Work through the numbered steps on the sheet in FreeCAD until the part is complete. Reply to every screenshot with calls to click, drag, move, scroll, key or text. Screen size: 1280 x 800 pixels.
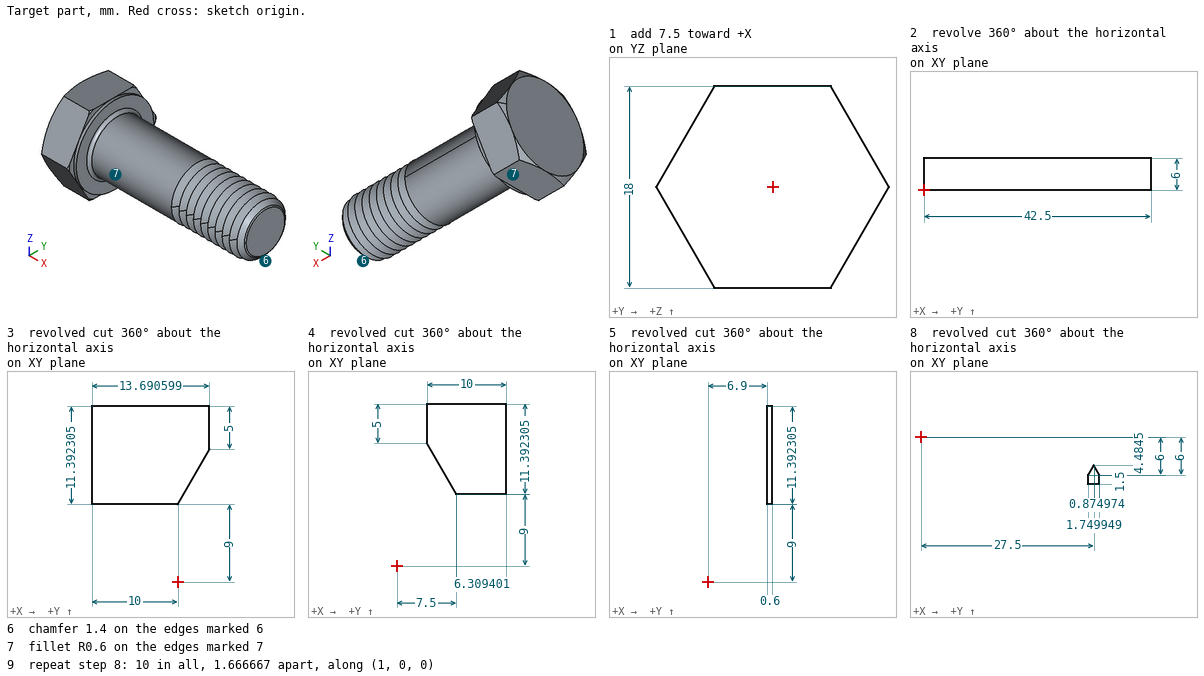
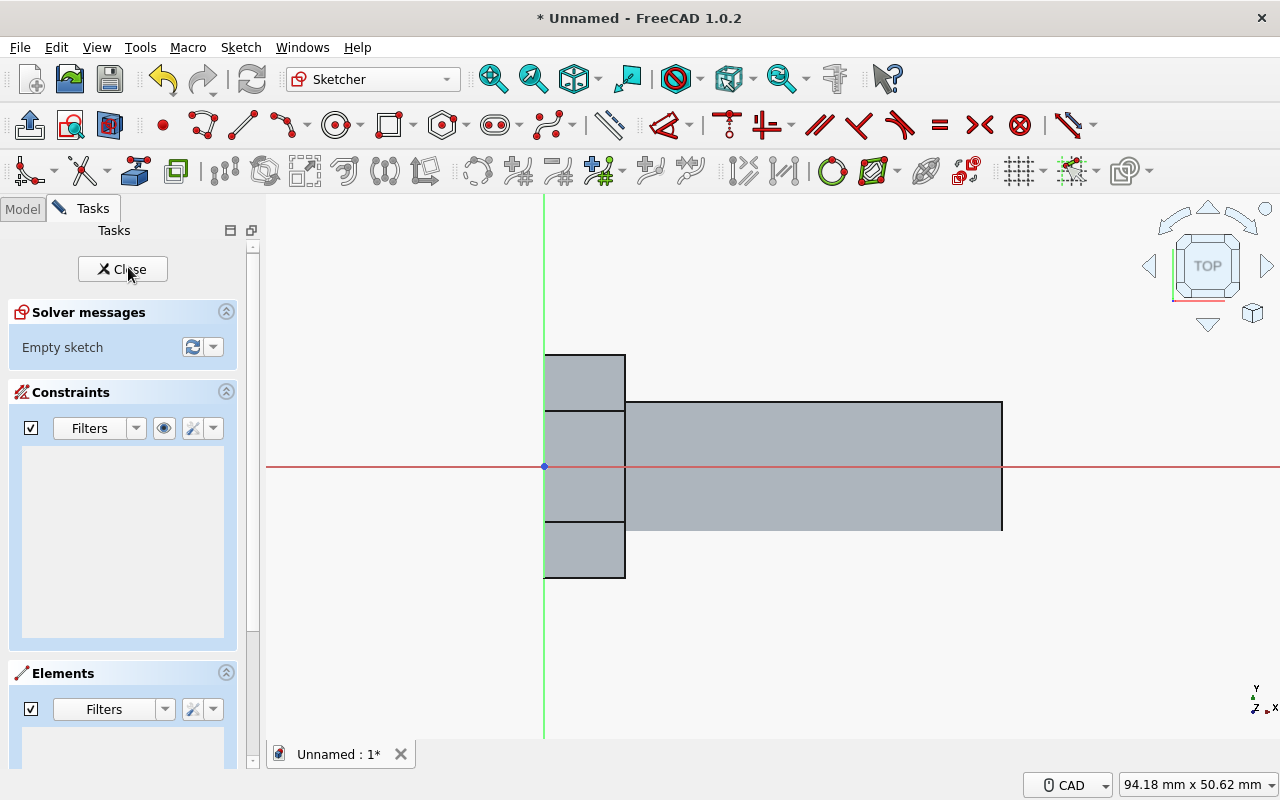
scroll(294, 222, up, 2)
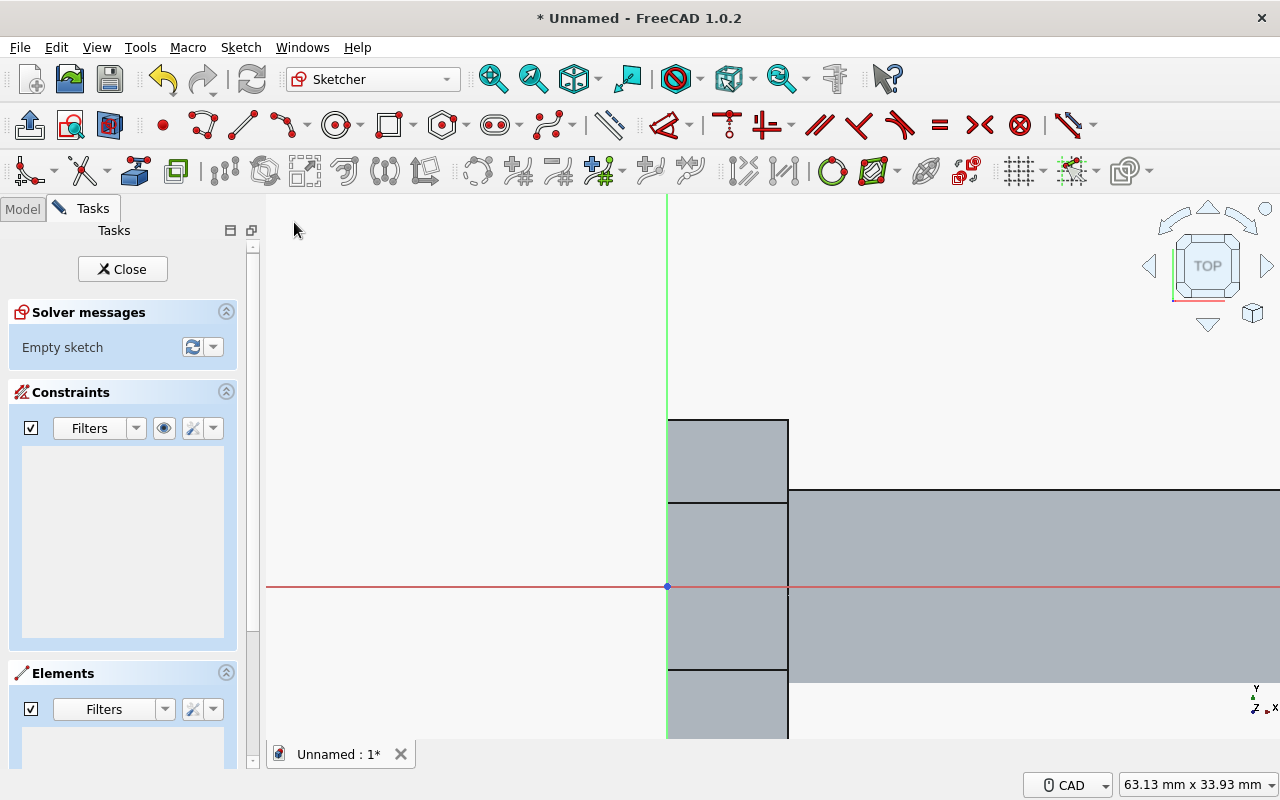
click(204, 126)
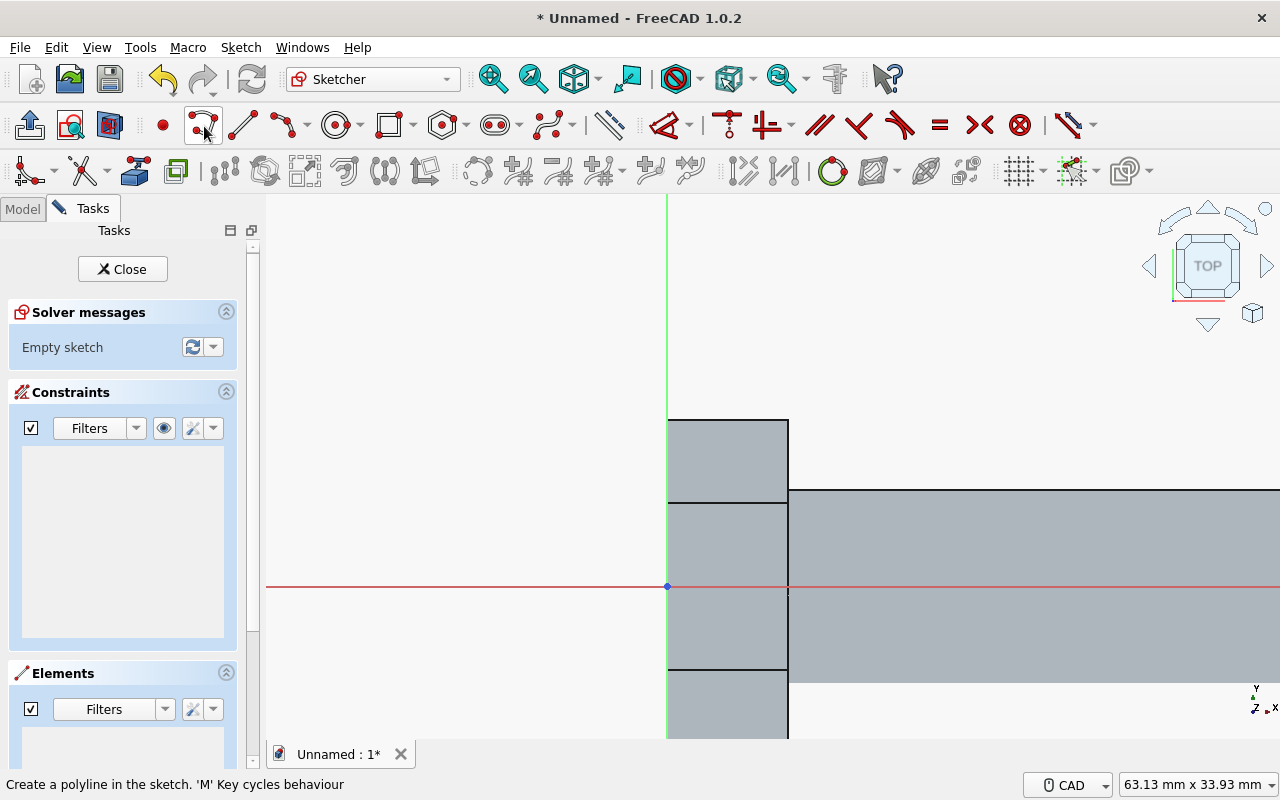
click(667, 442)
click(727, 339)
click(727, 259)
click(507, 259)
click(507, 442)
click(667, 443)
key(Escape)
key(Escape)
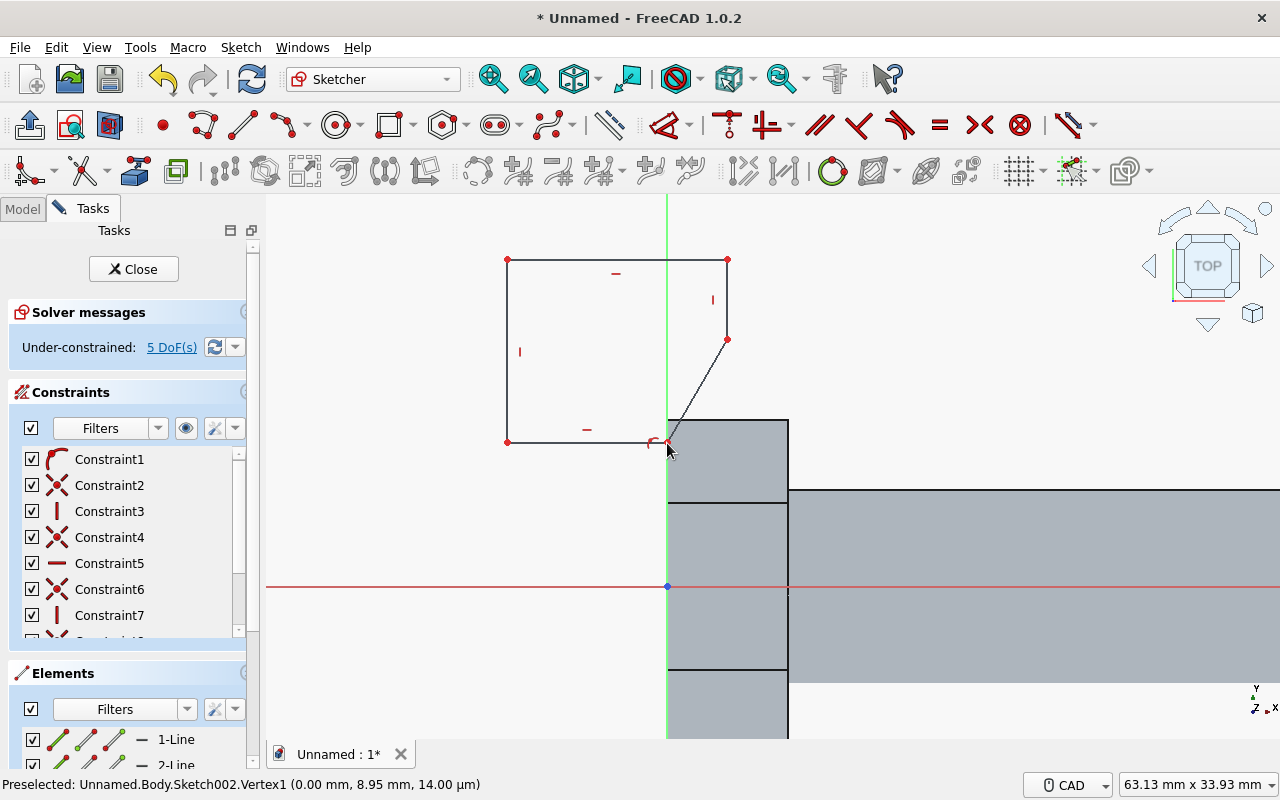
click(727, 316)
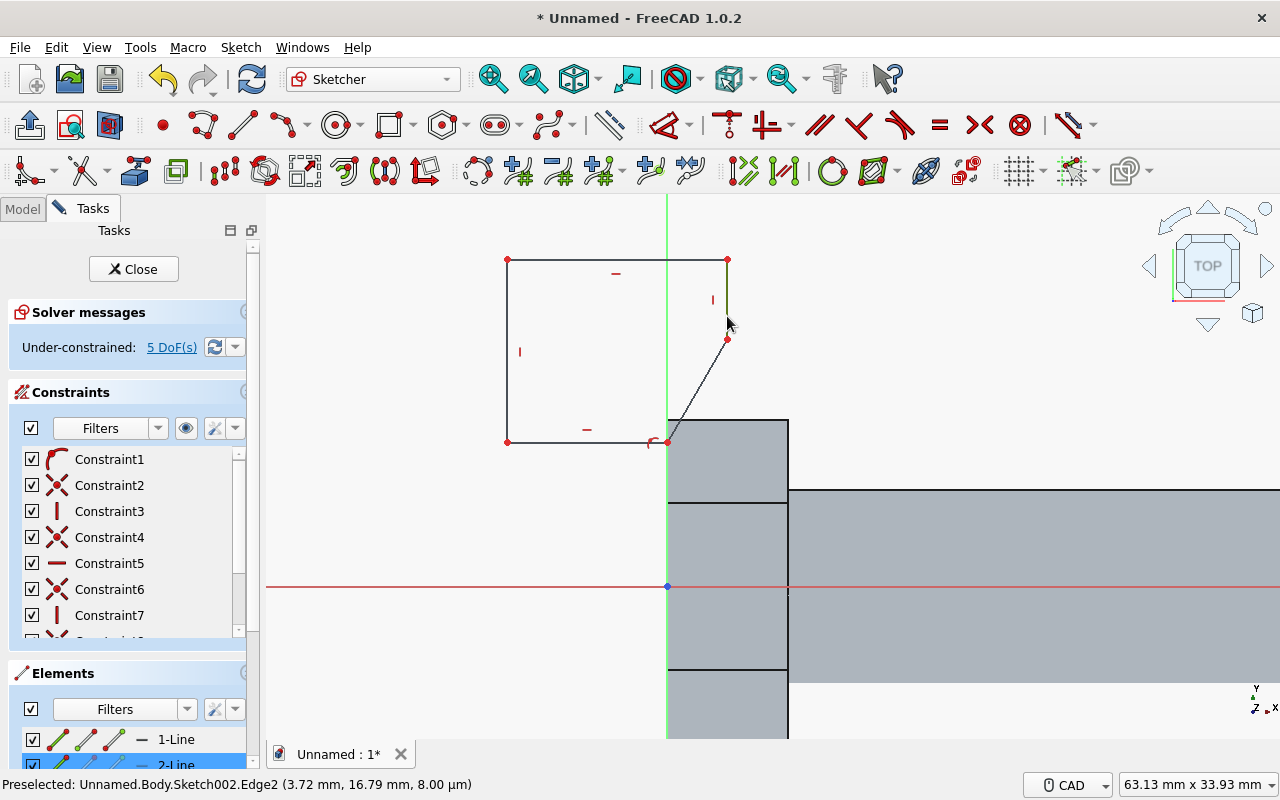
key(i)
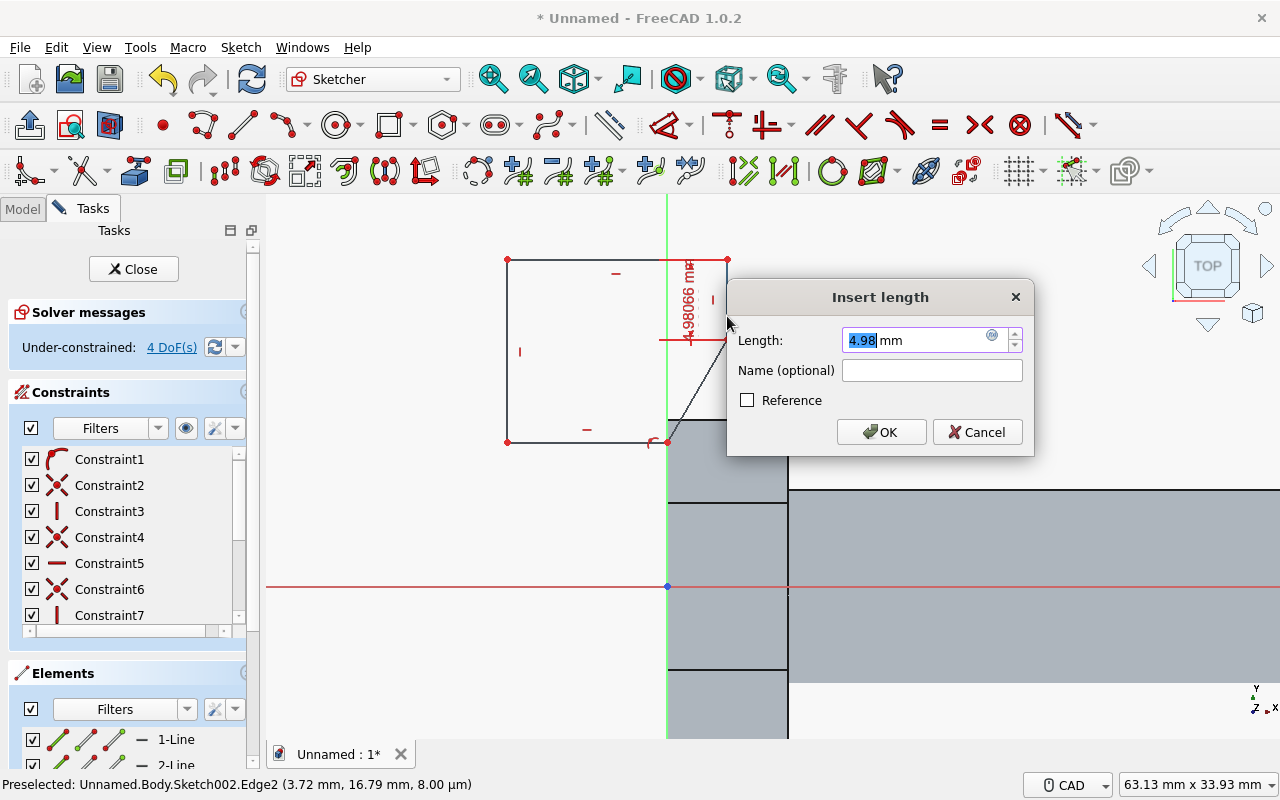
text(5)
key(Return)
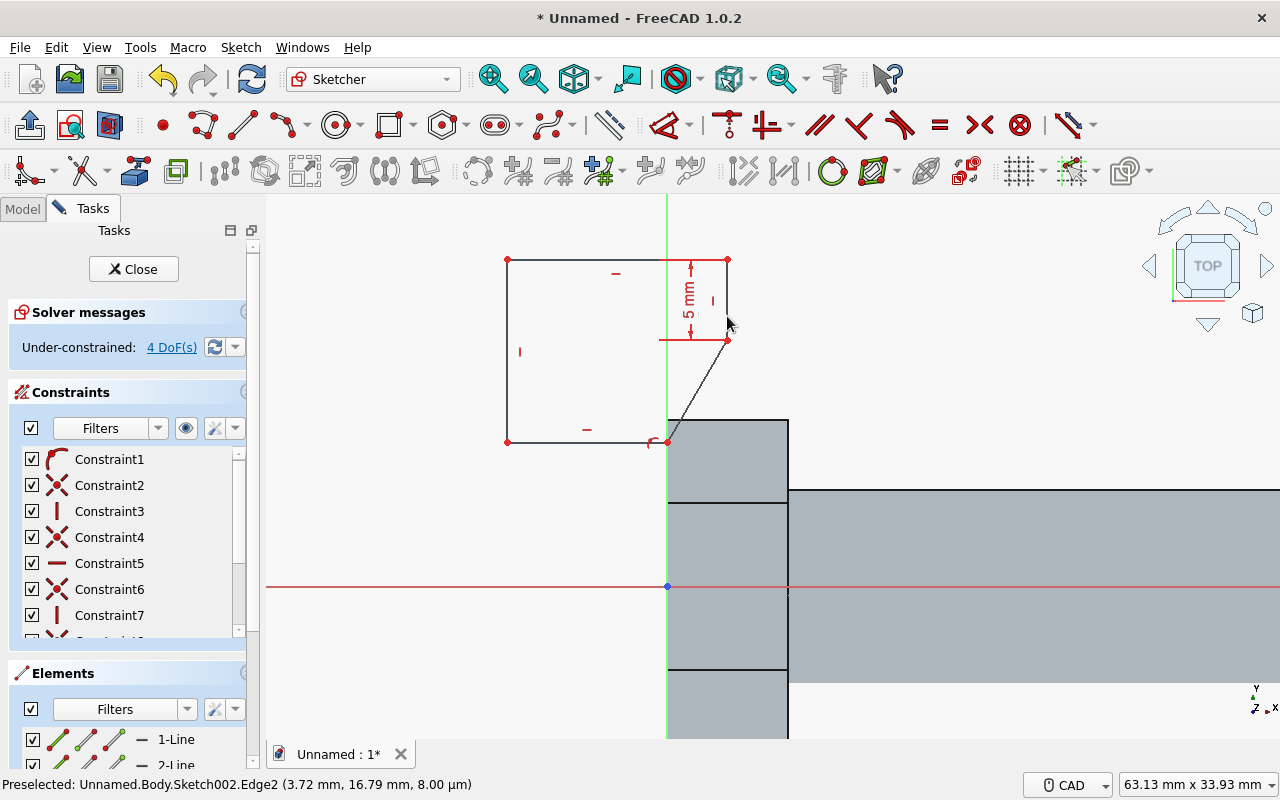
click(555, 443)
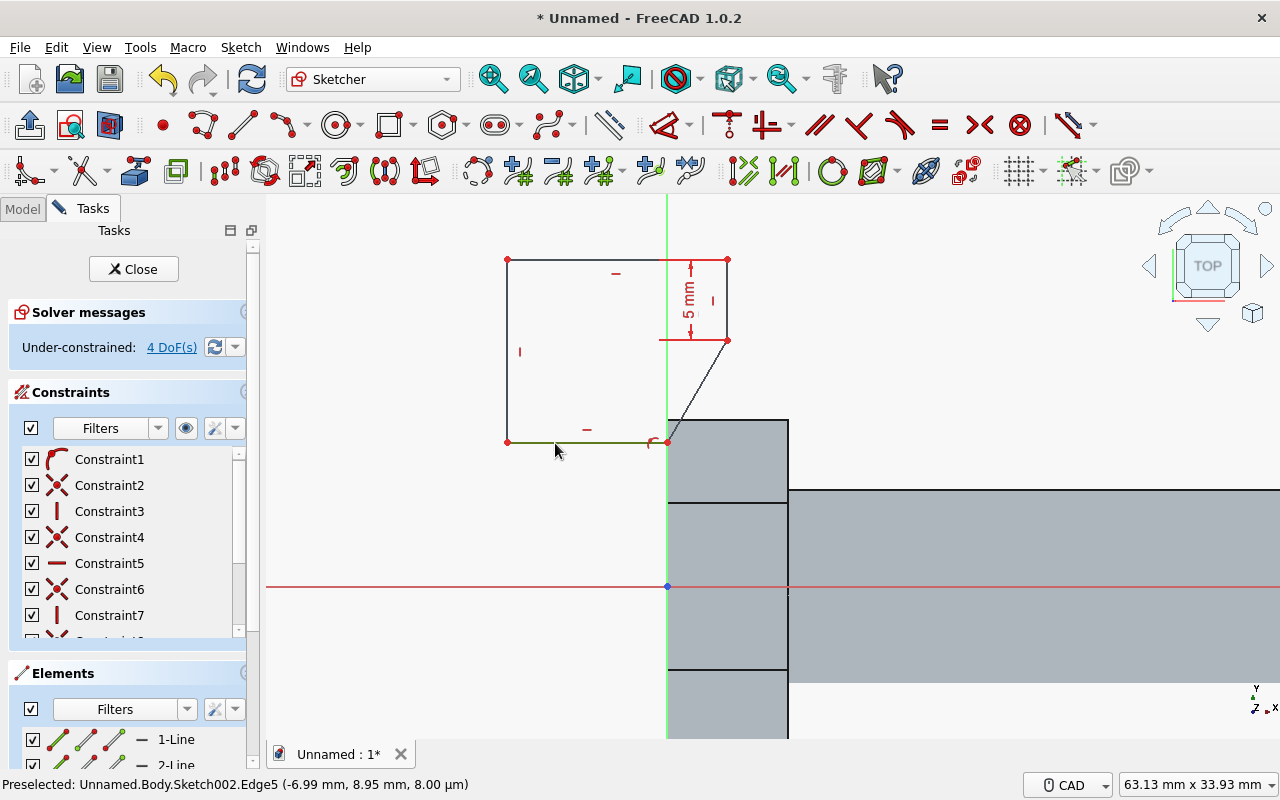
key(l)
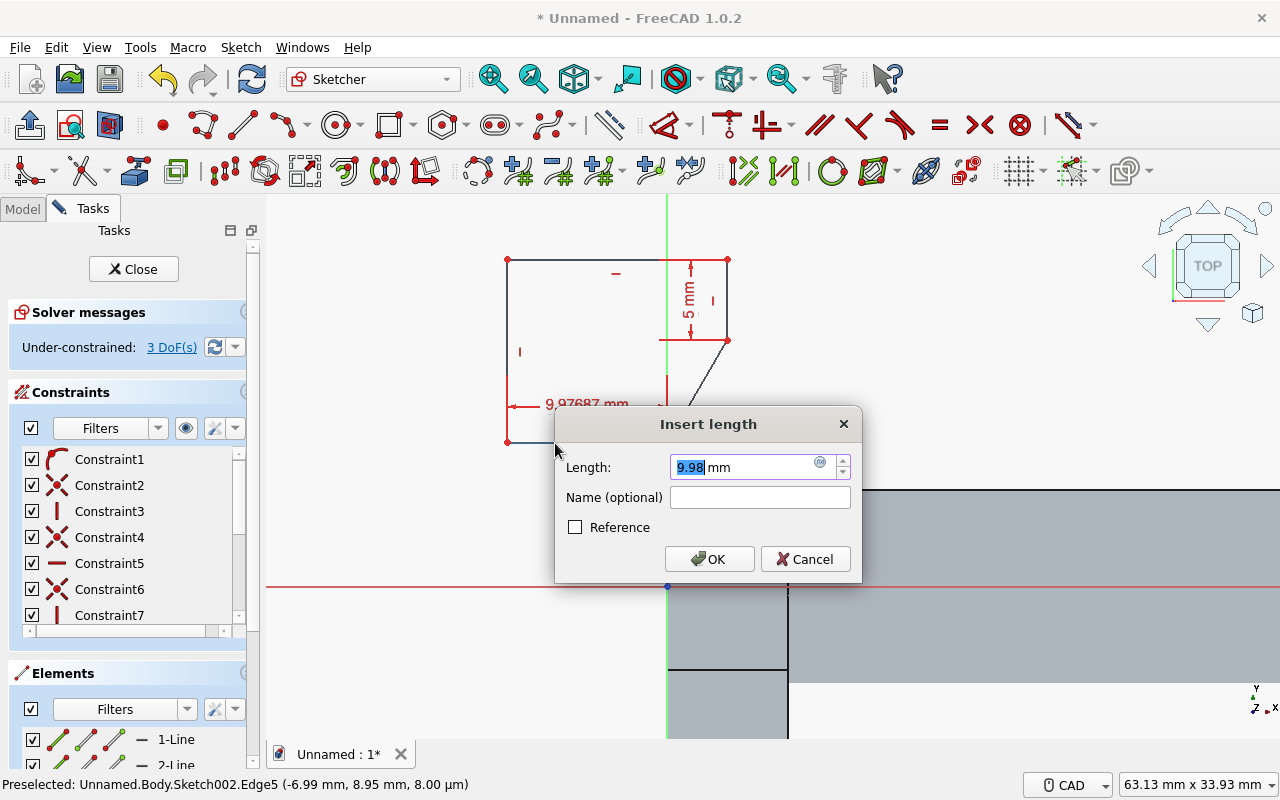
text(10)
key(Return)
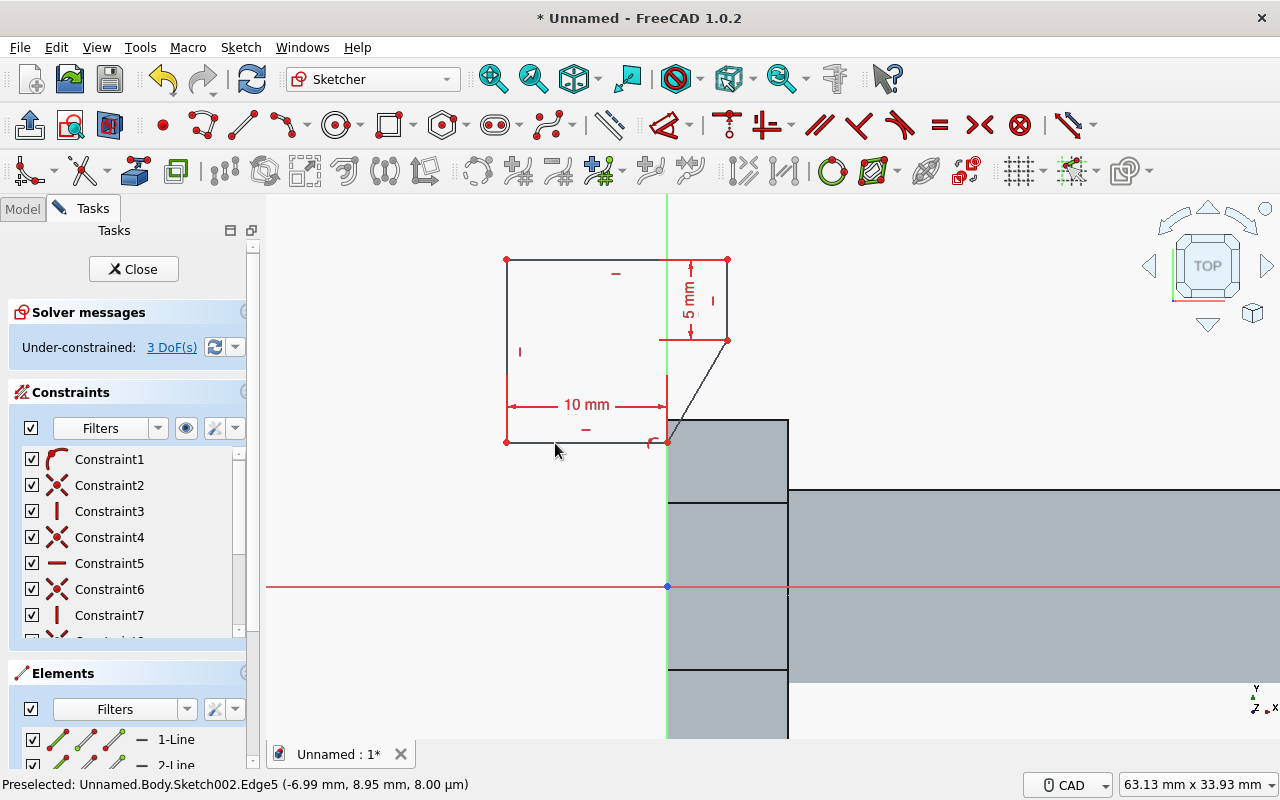
click(667, 443)